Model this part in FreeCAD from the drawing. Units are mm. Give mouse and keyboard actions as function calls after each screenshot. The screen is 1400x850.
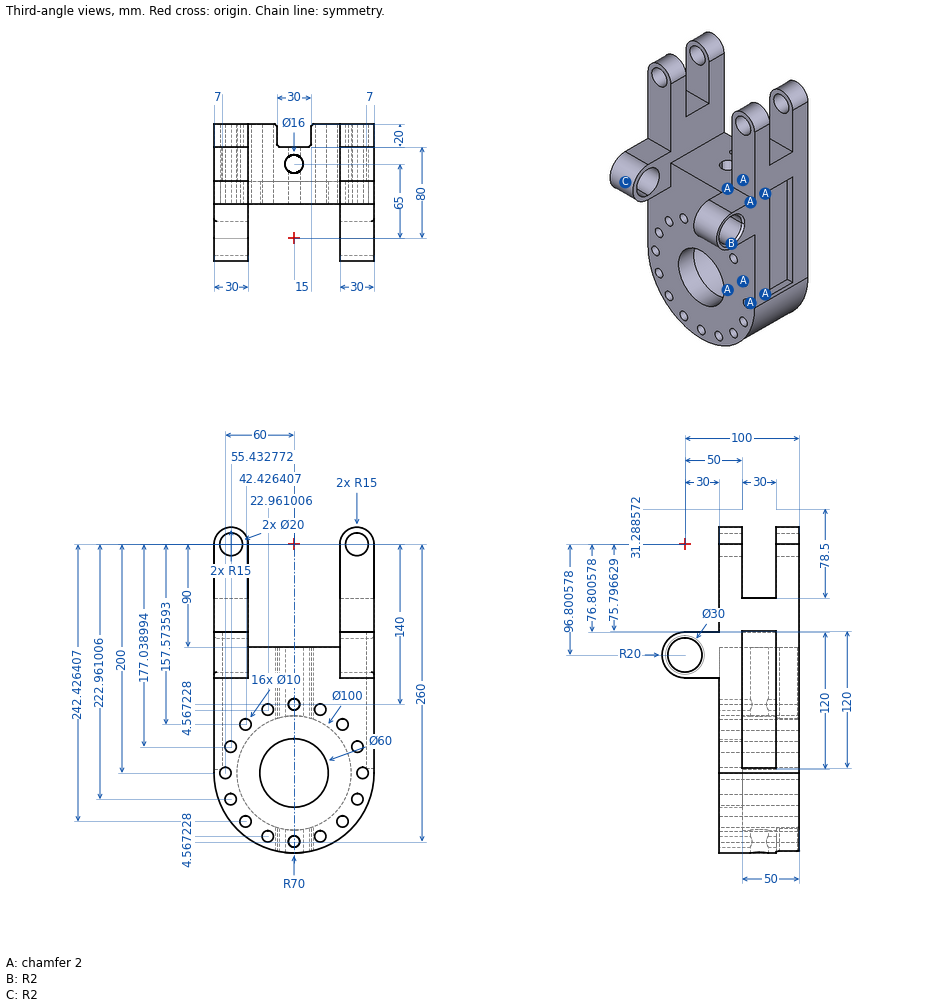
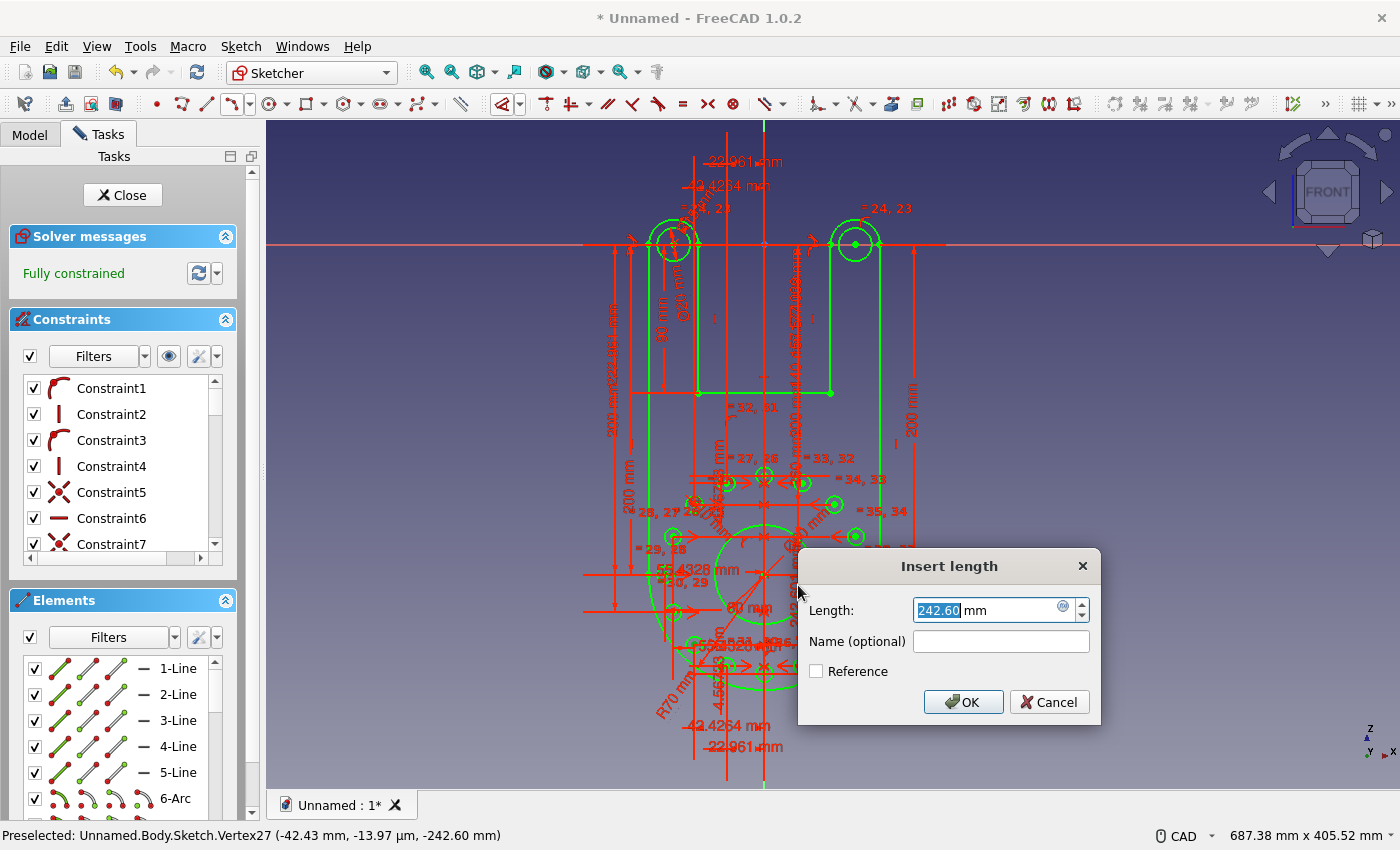
text(242.426407)
key(Return)
key(Escape)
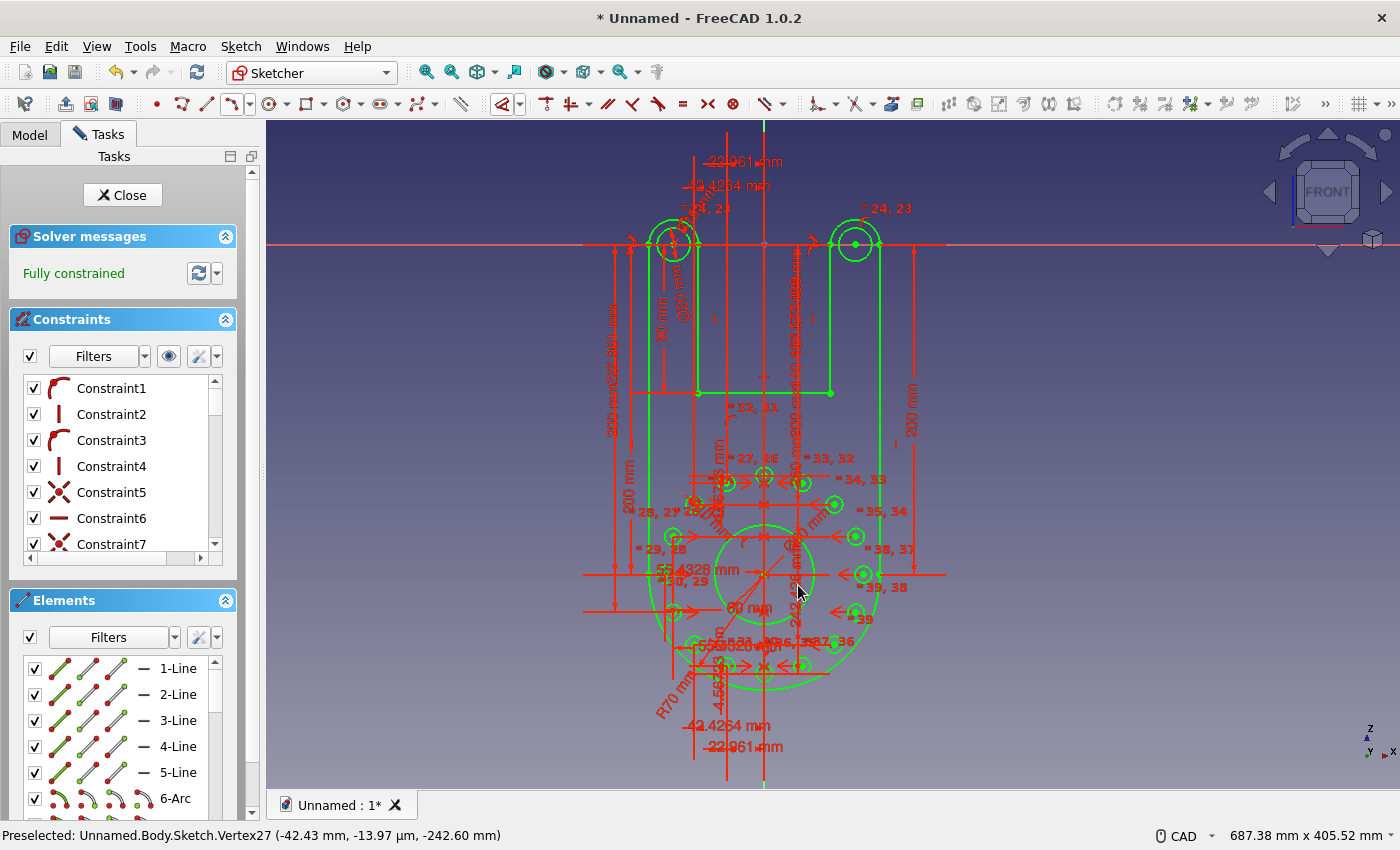
click(123, 195)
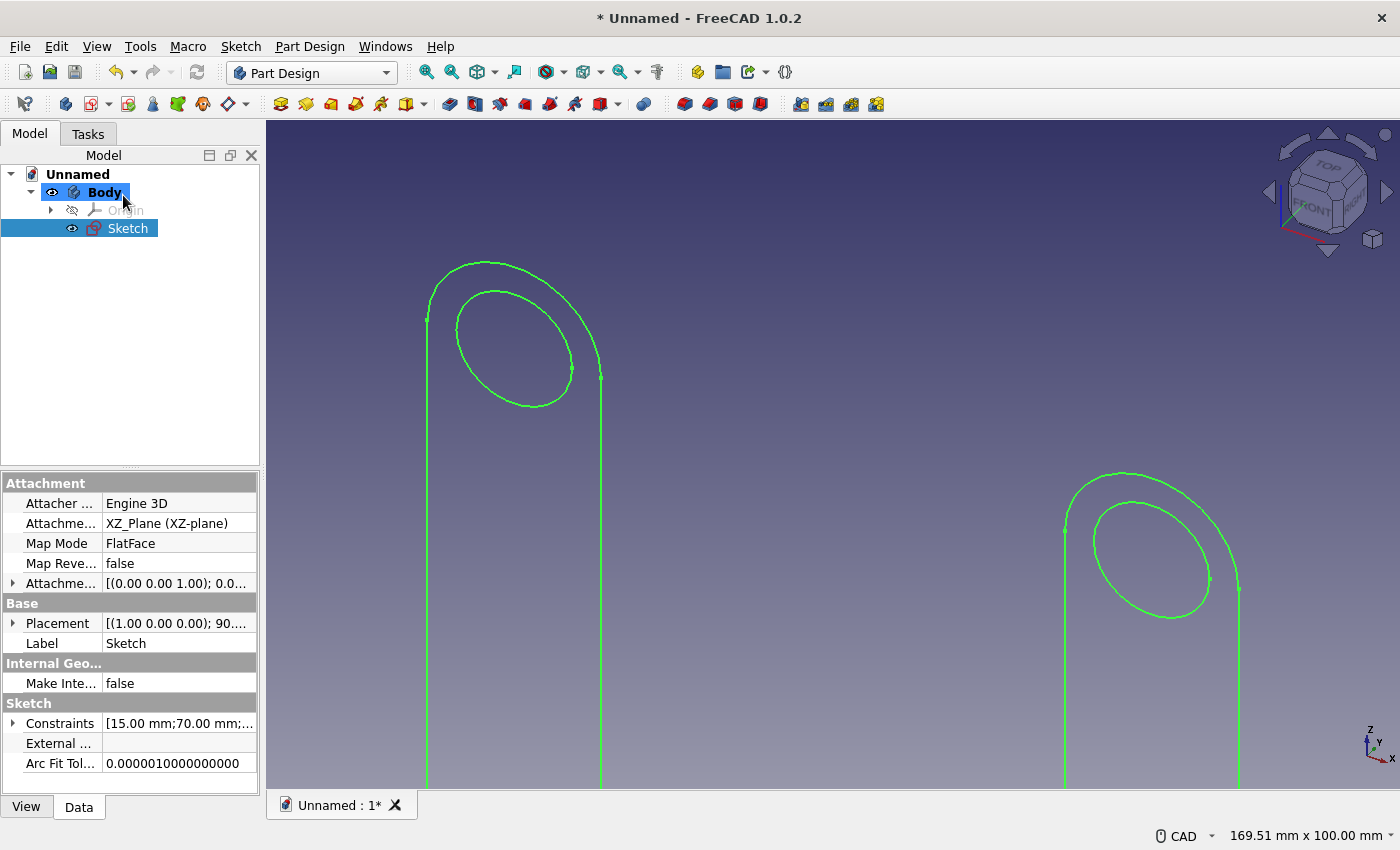
click(281, 104)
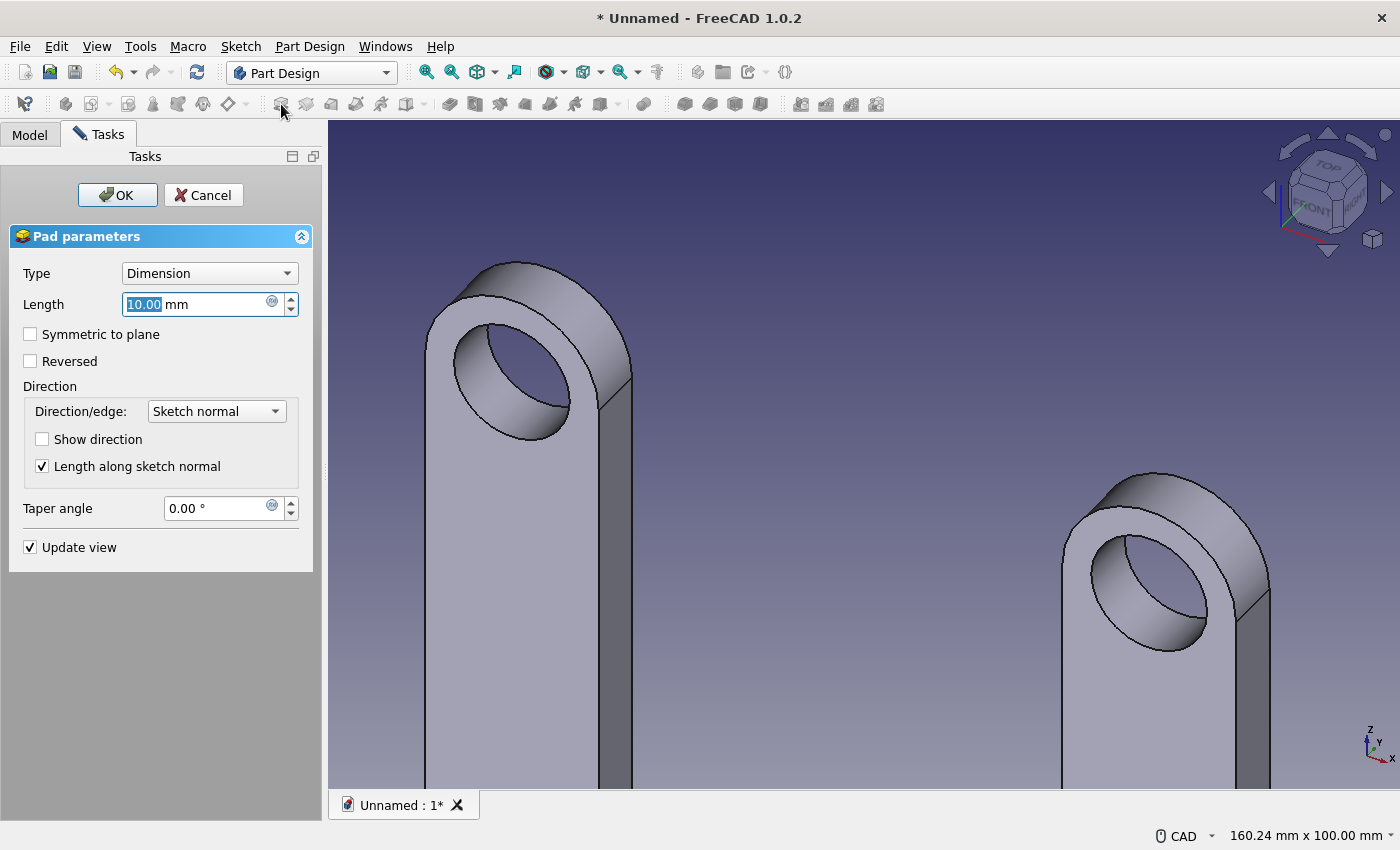
text(100)
key(Tab)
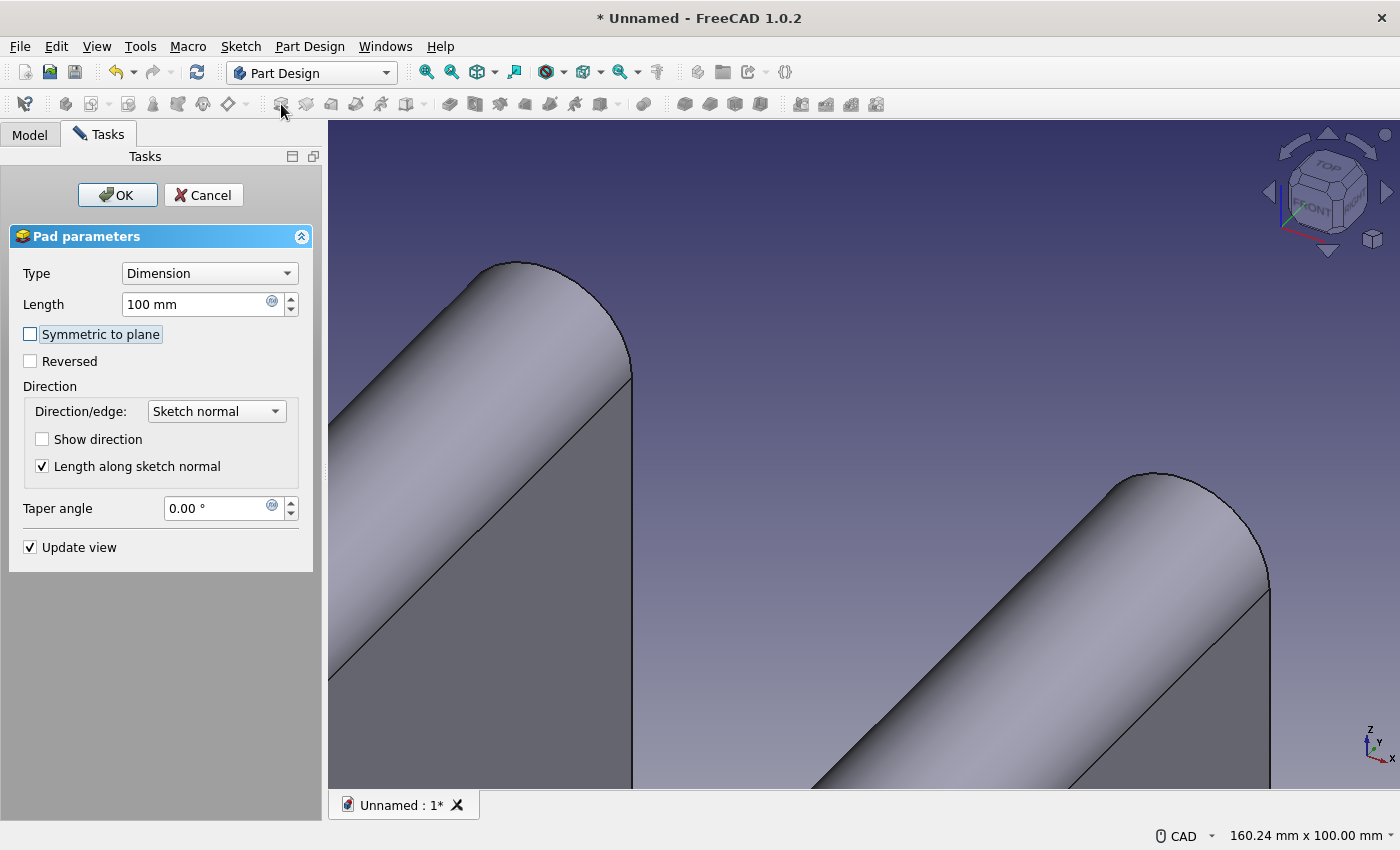
click(31, 361)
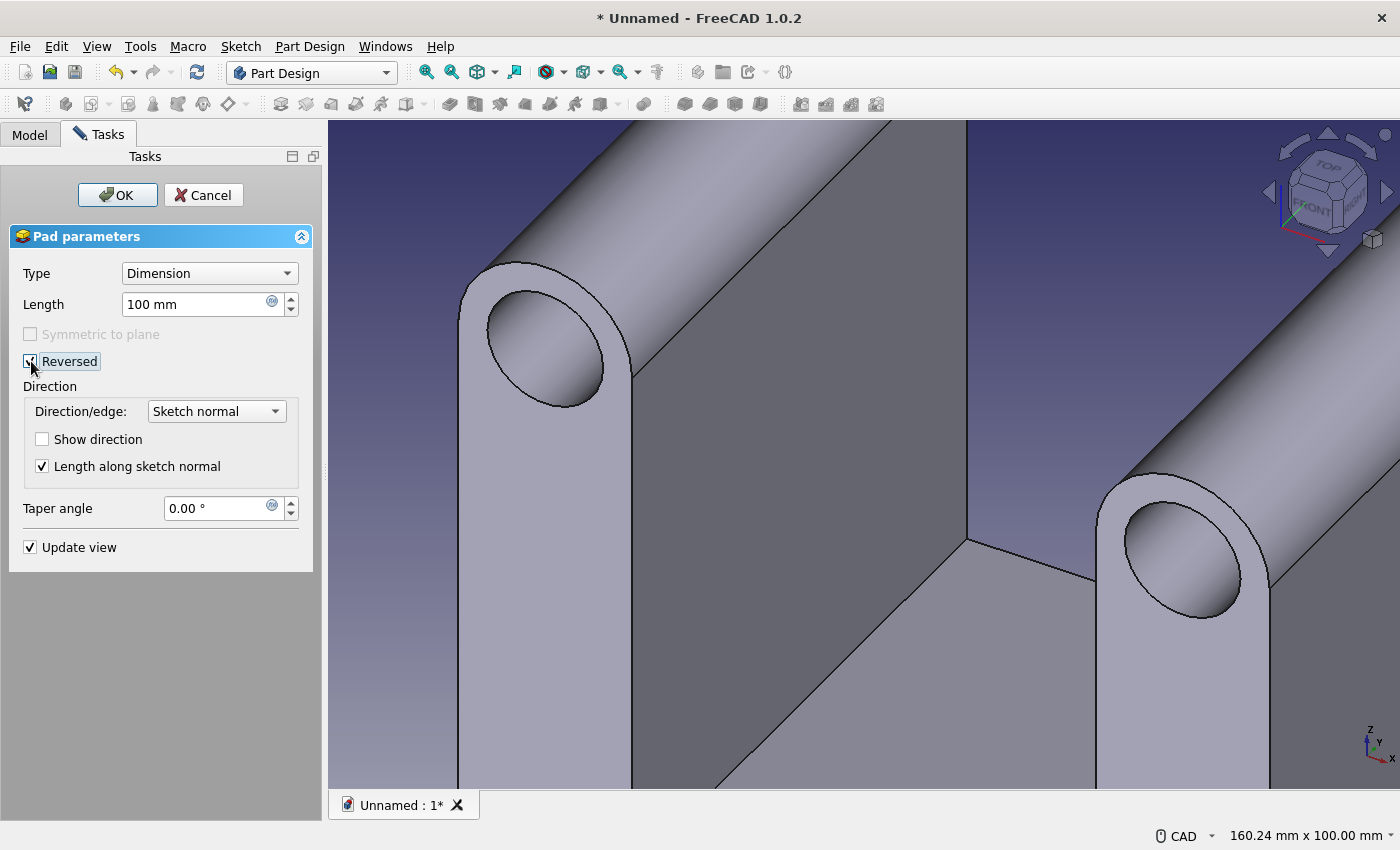
click(118, 195)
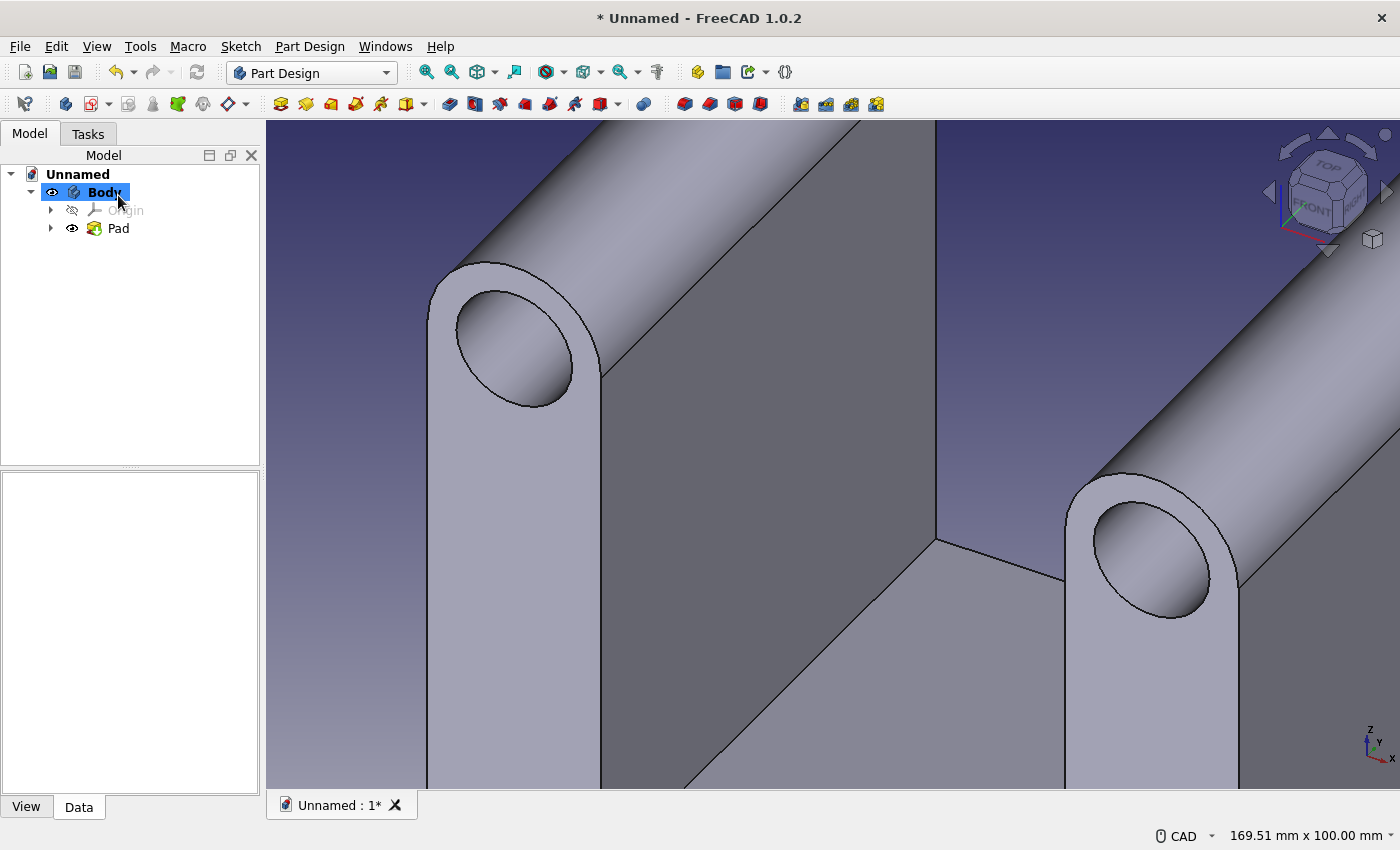
key(v)
key(f)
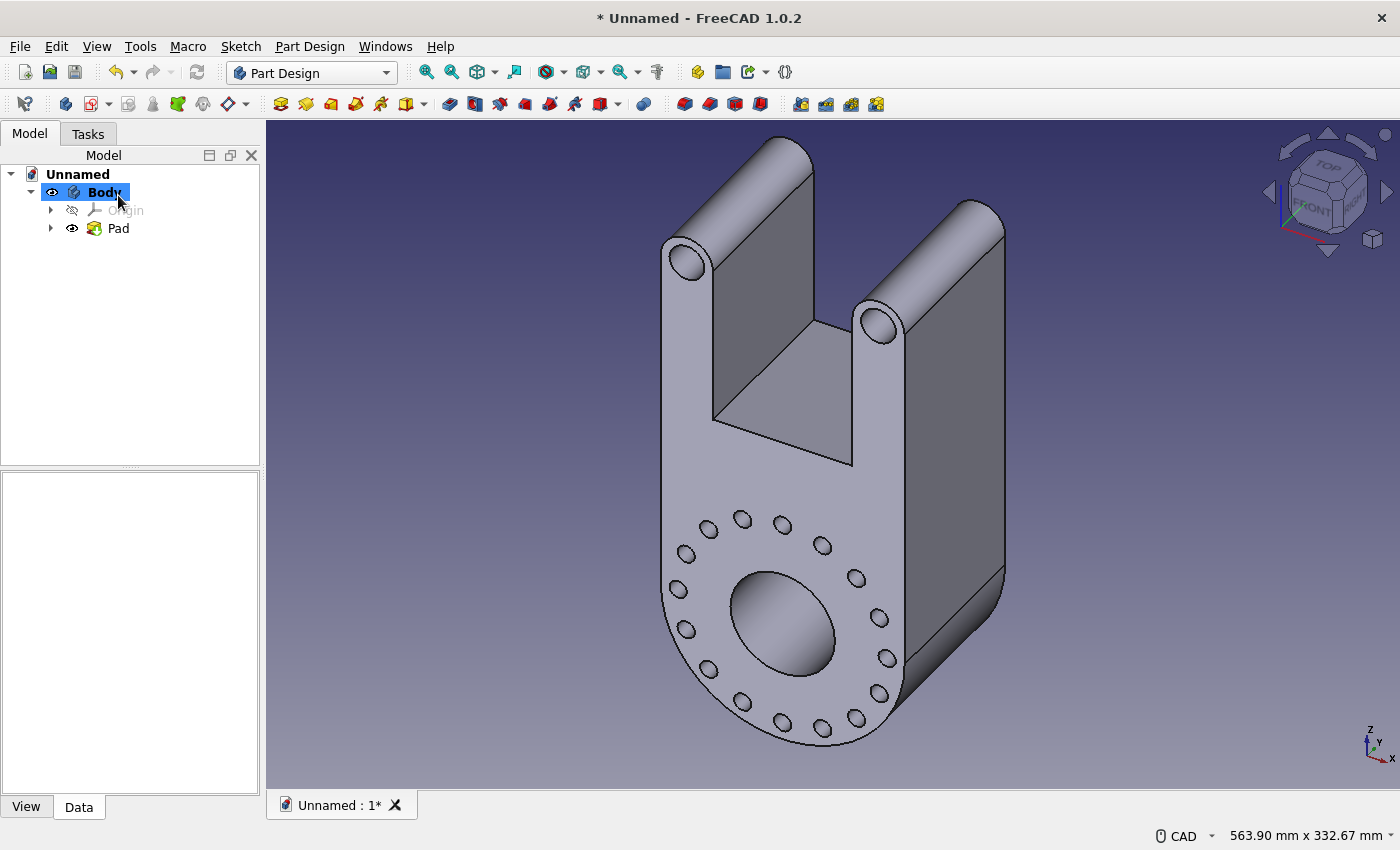
click(833, 392)